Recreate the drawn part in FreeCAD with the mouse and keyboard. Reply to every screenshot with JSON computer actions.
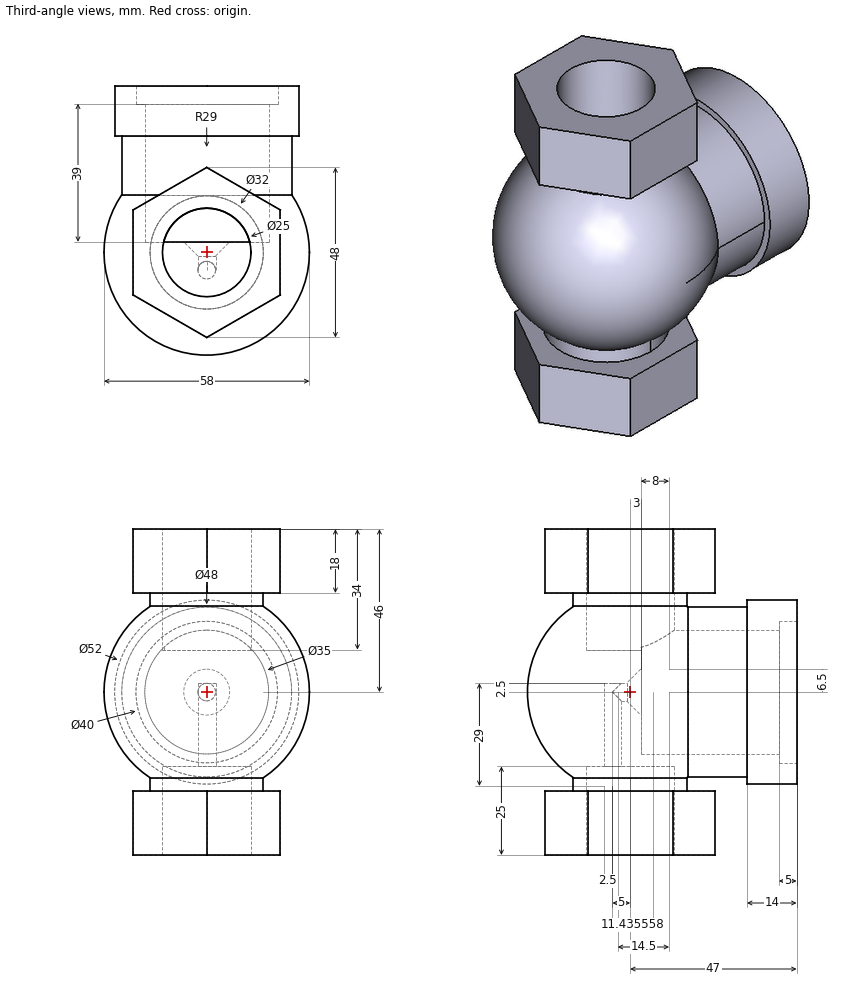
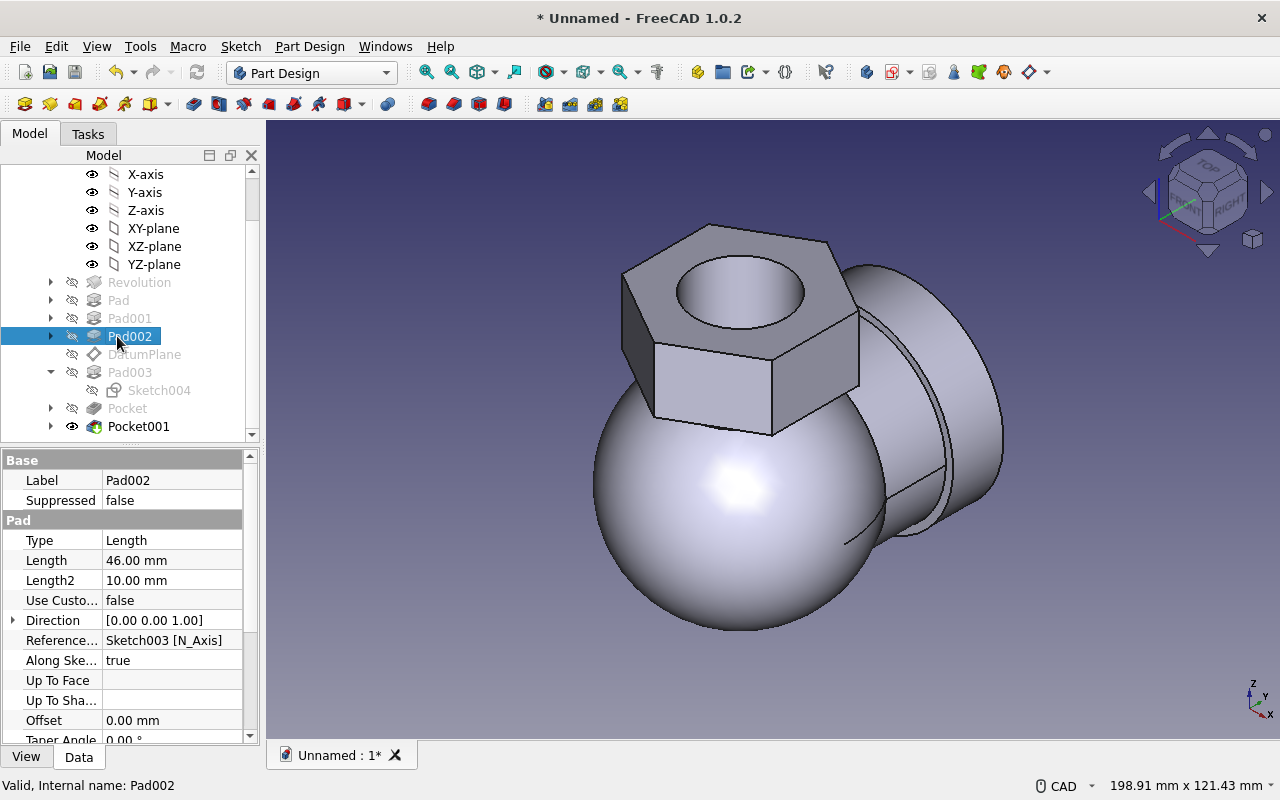
{"action": "left_click", "coordinate": [117, 372], "text": "ctrl"}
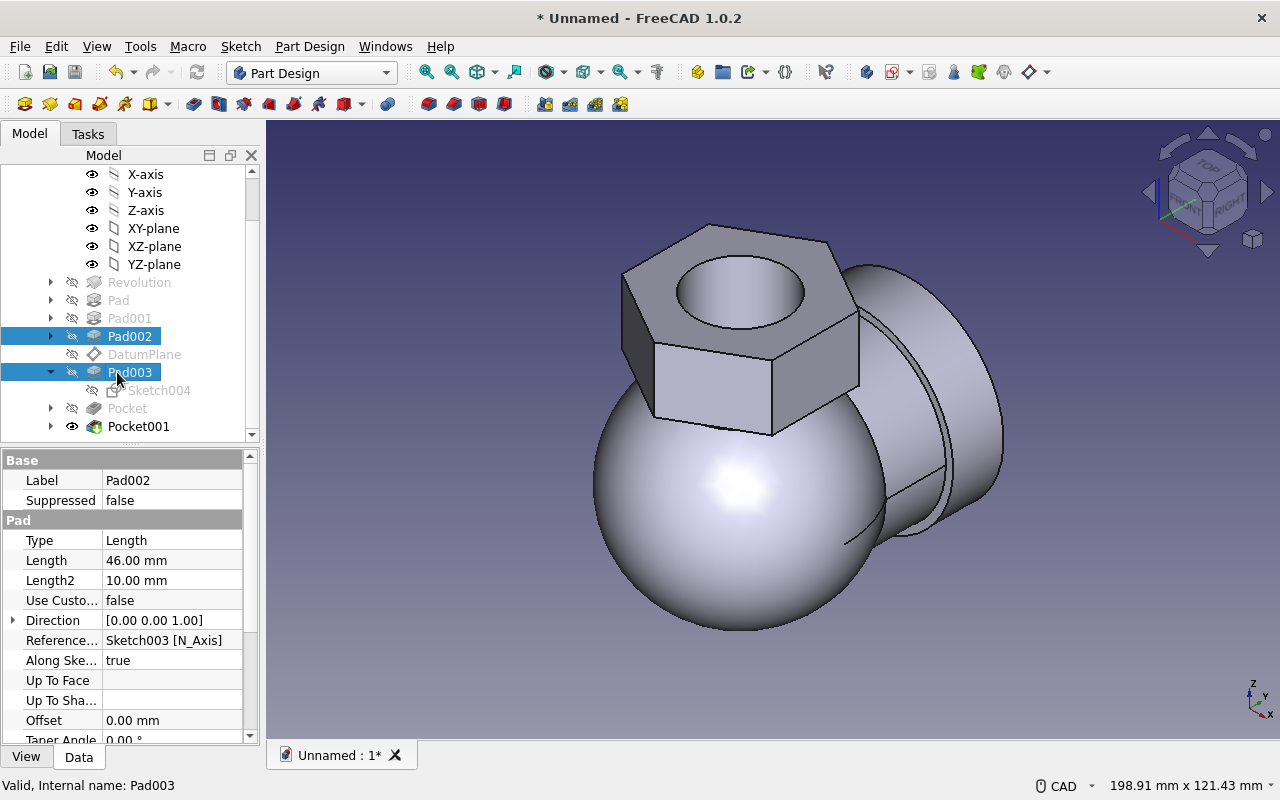
{"action": "left_click", "coordinate": [545, 104]}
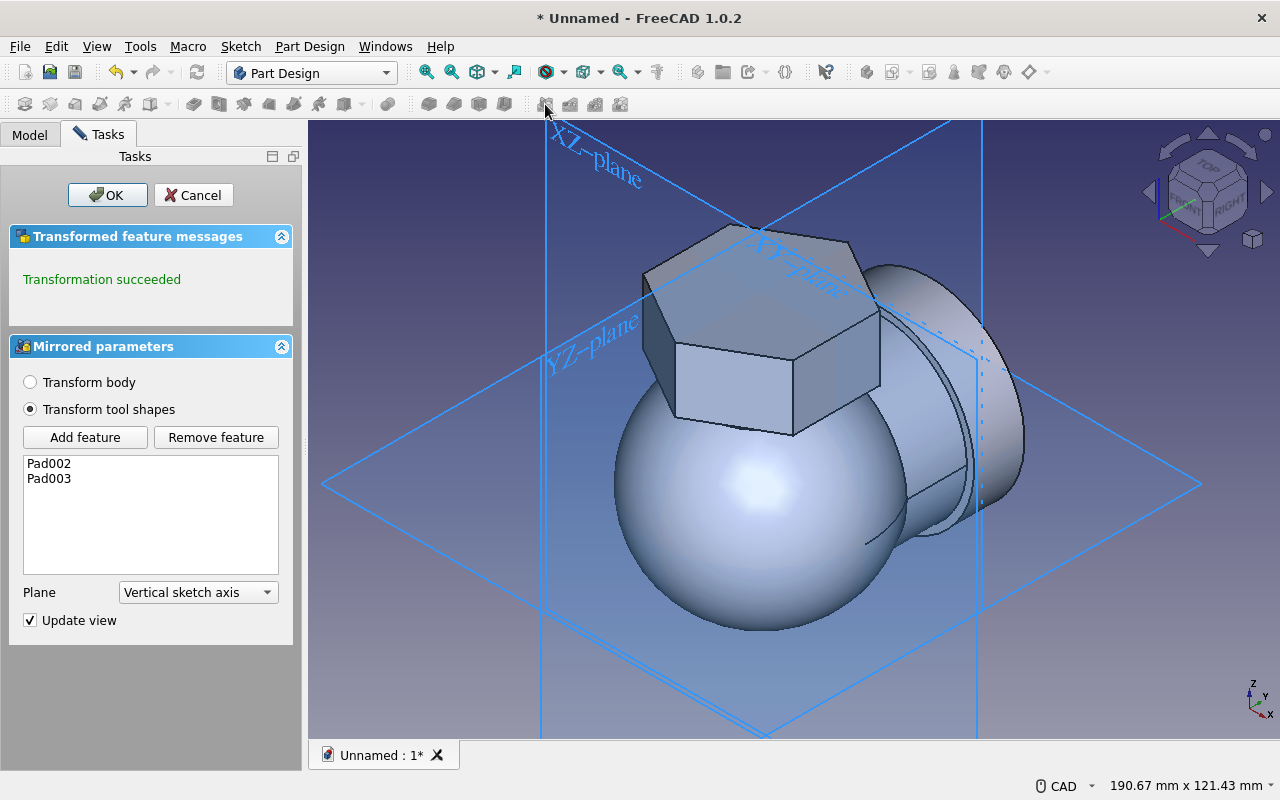
{"action": "left_click", "coordinate": [199, 592]}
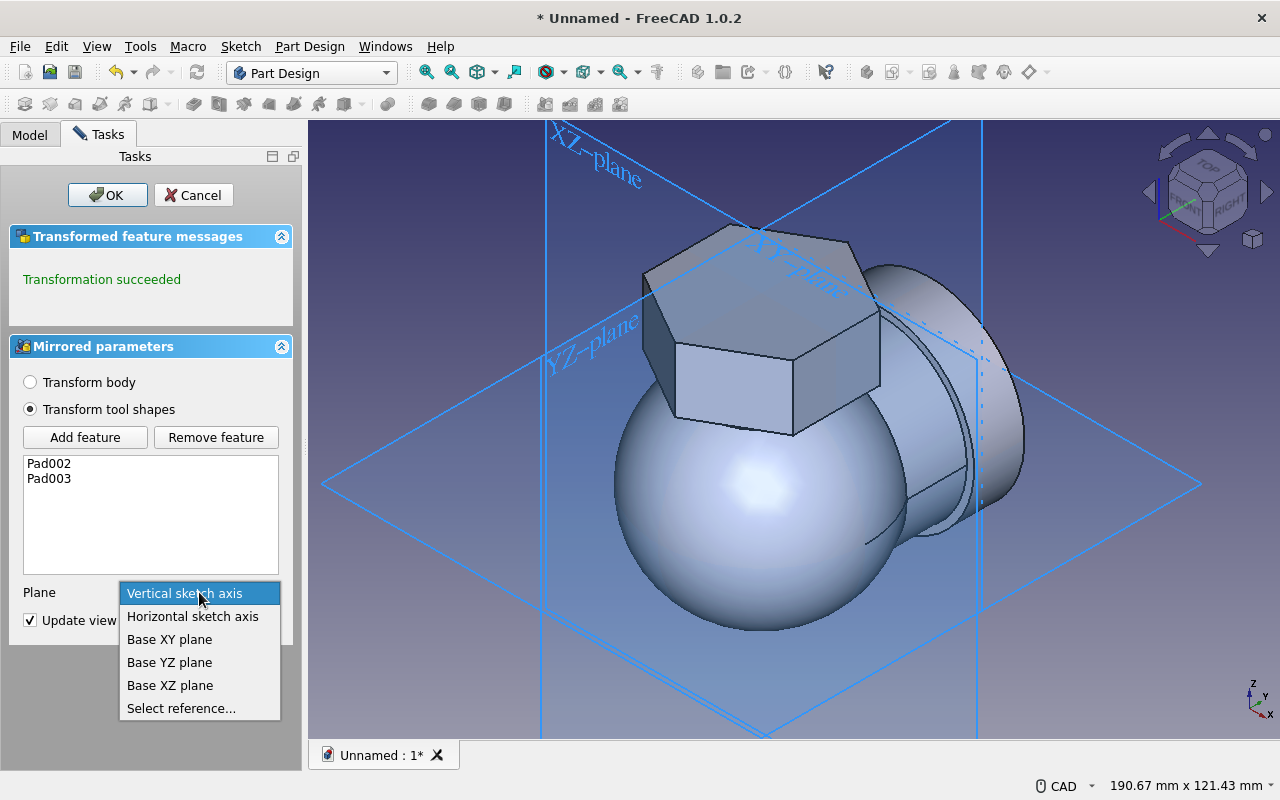
{"action": "left_click", "coordinate": [198, 640]}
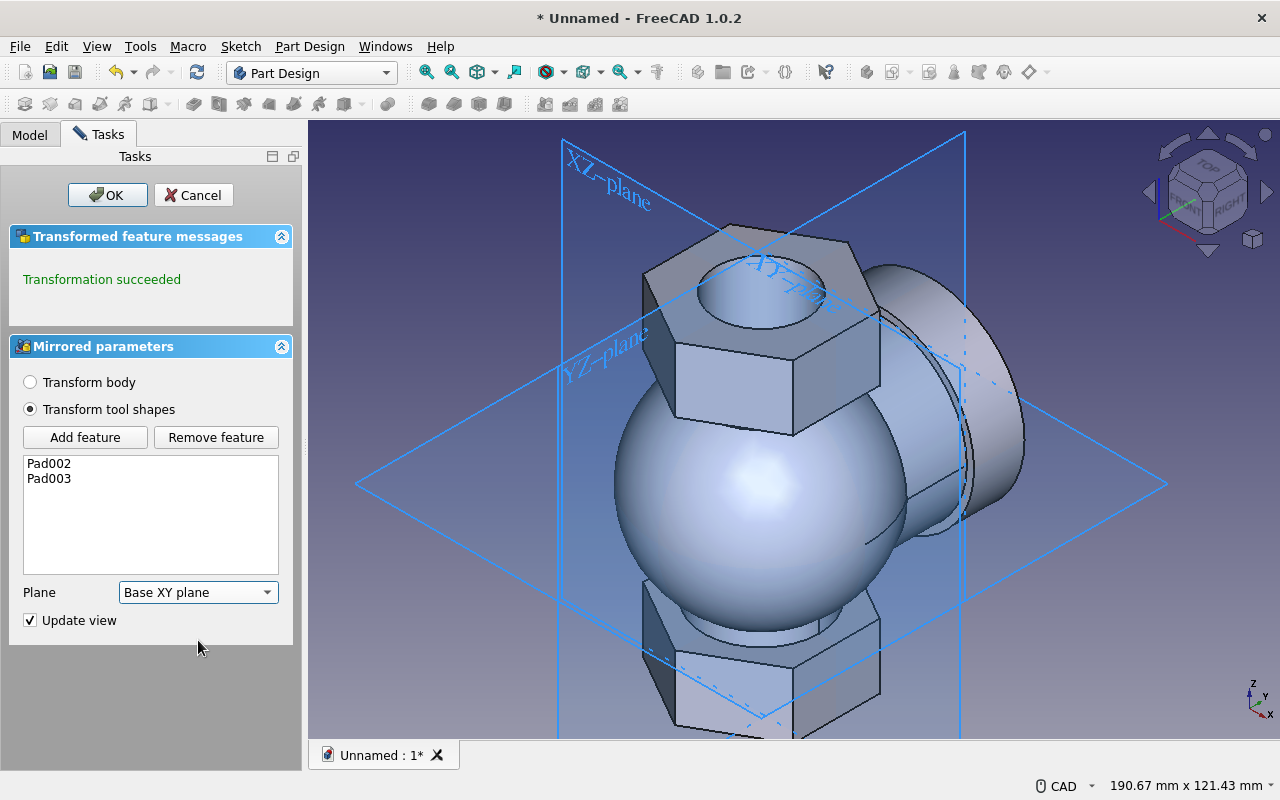
{"action": "left_click", "coordinate": [108, 195]}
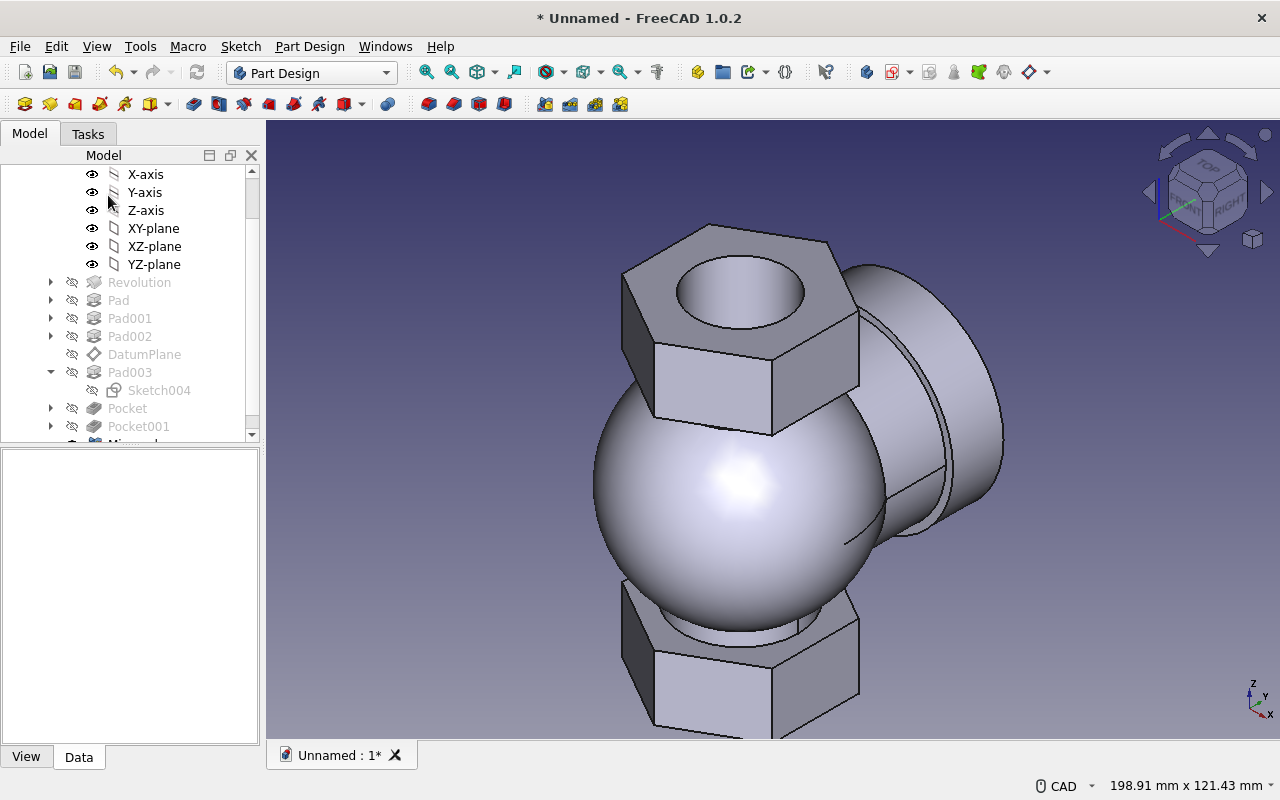
{"action": "left_click", "coordinate": [427, 72]}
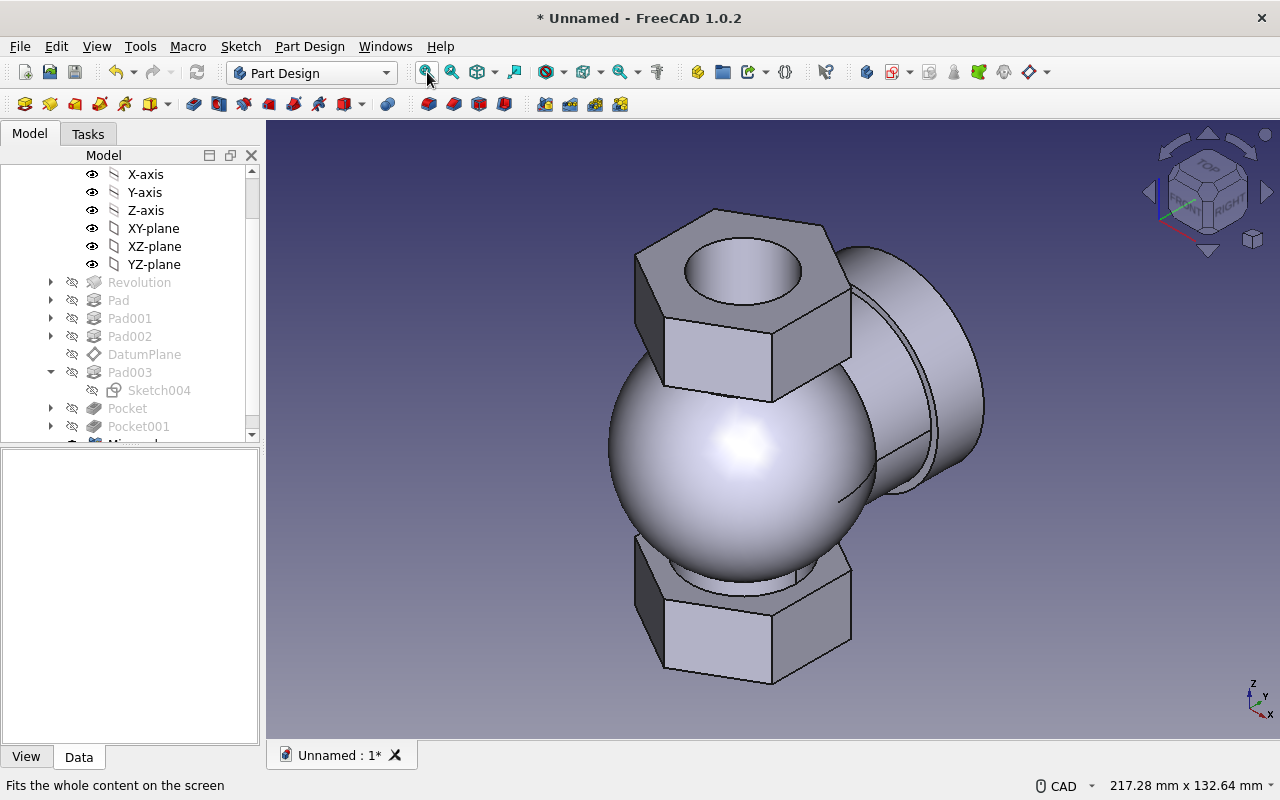
{"action": "scroll", "coordinate": [161, 296], "scroll_direction": "down", "scroll_amount": 3}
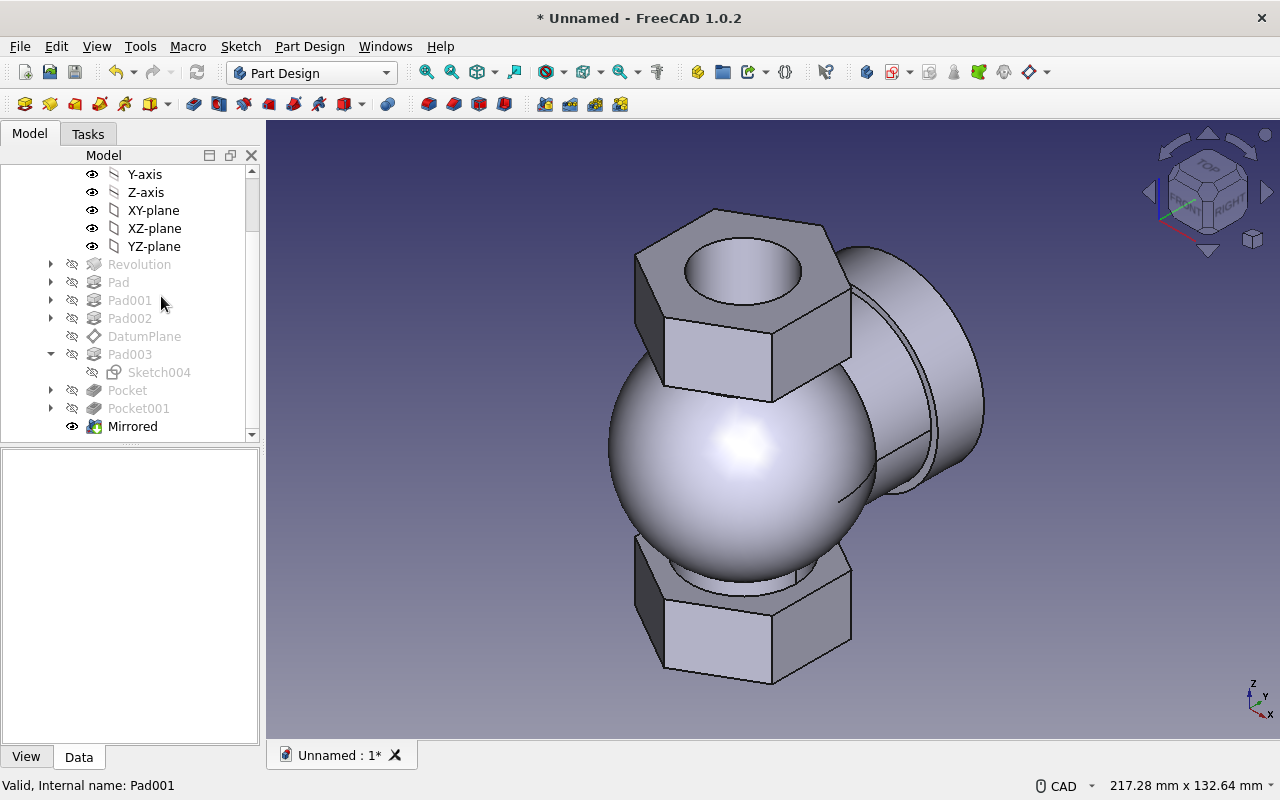
{"action": "scroll", "coordinate": [161, 296], "scroll_direction": "up", "scroll_amount": 15}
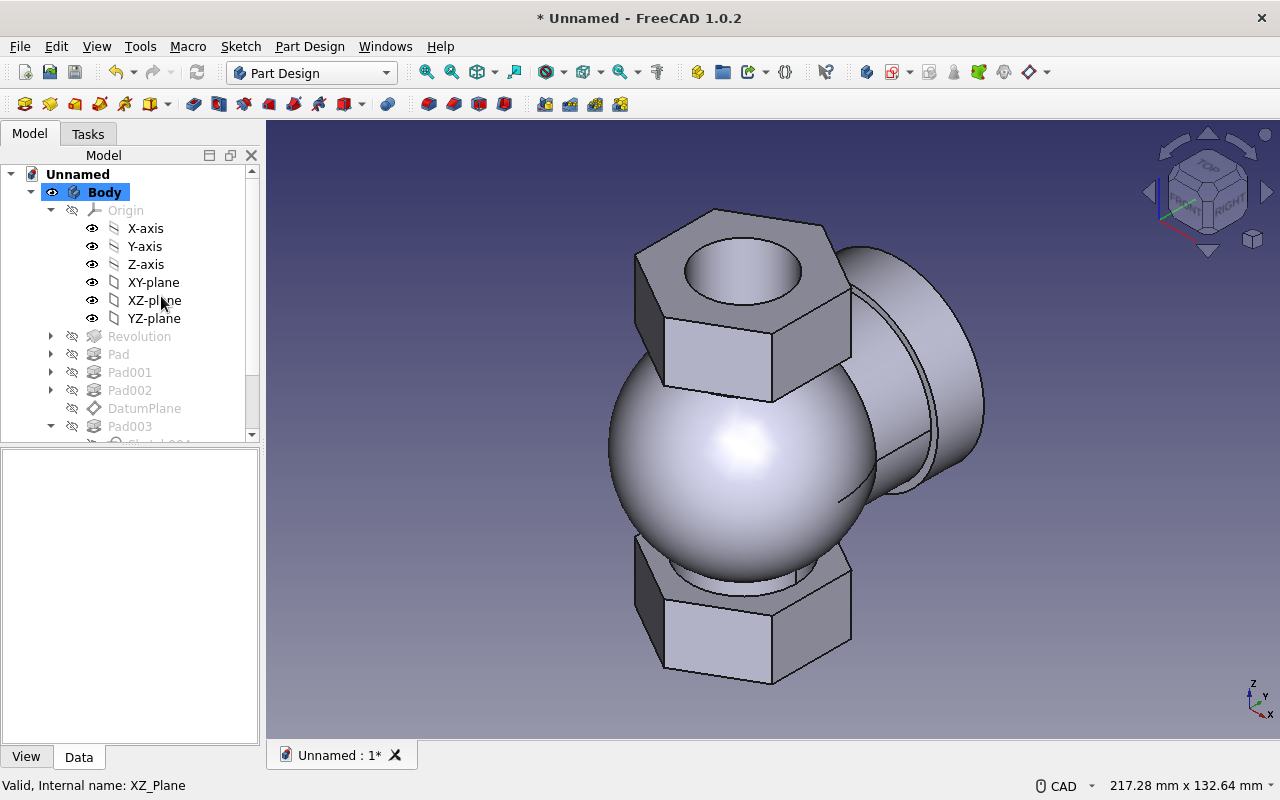
{"action": "left_click", "coordinate": [137, 282]}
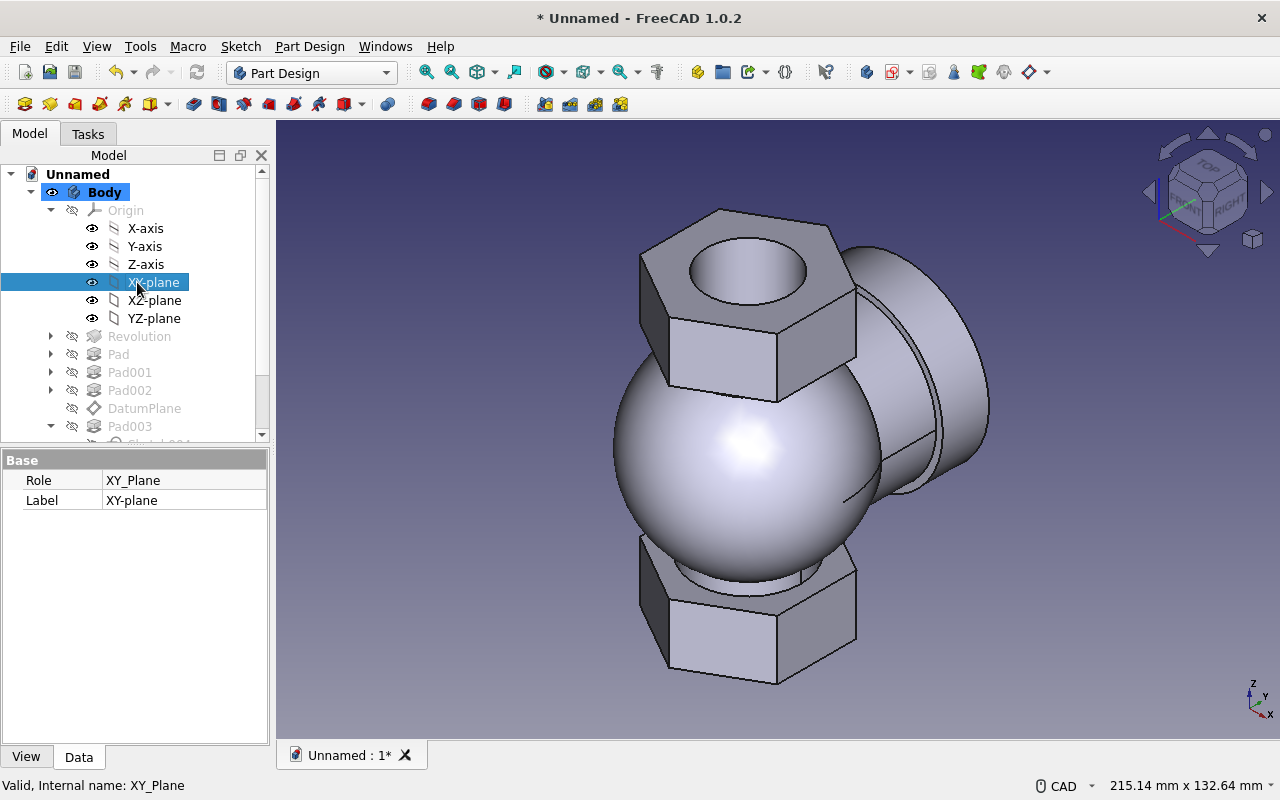
{"action": "left_click", "coordinate": [1028, 72]}